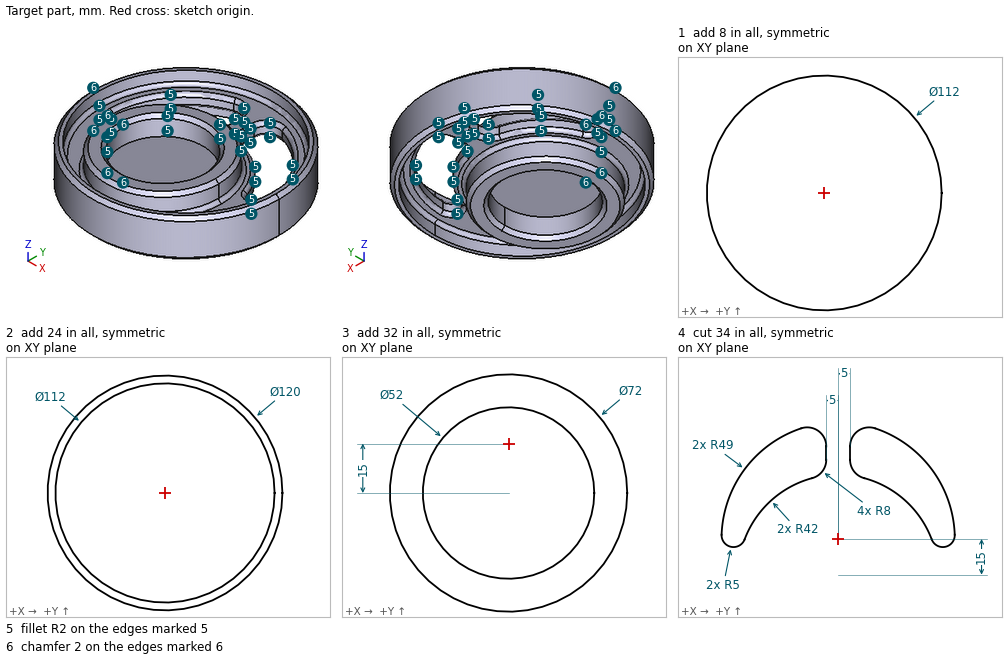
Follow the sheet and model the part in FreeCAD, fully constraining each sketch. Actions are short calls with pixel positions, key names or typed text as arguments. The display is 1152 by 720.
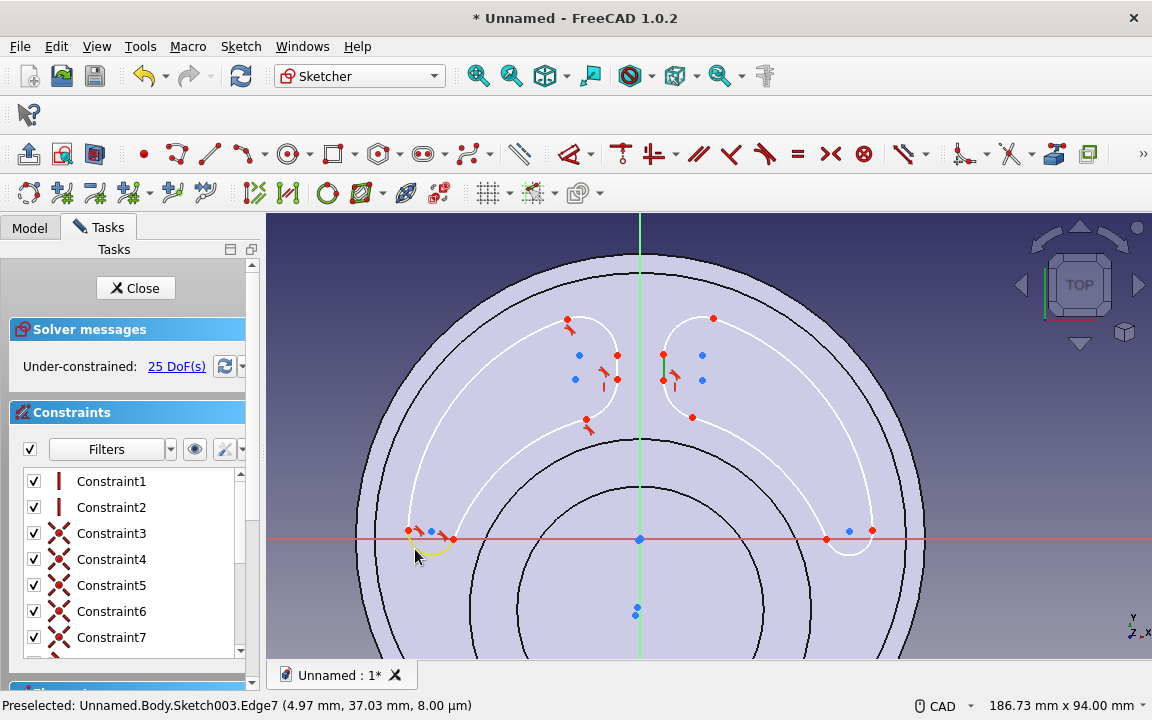
click(693, 318)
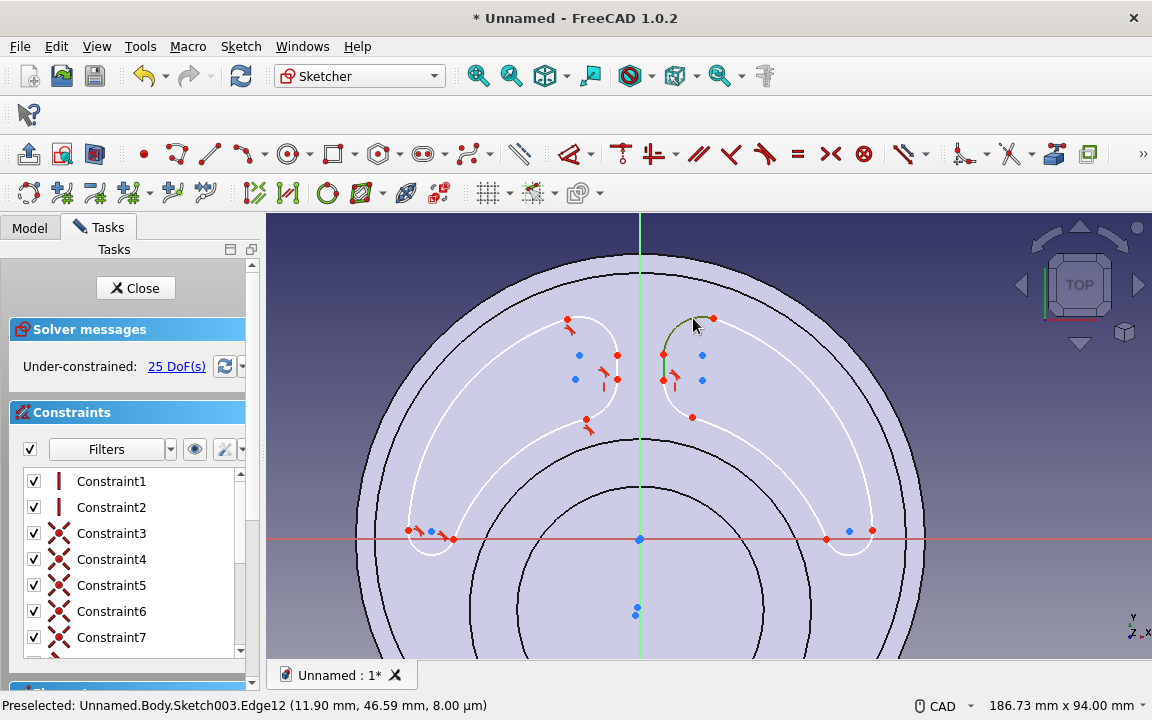
key(t)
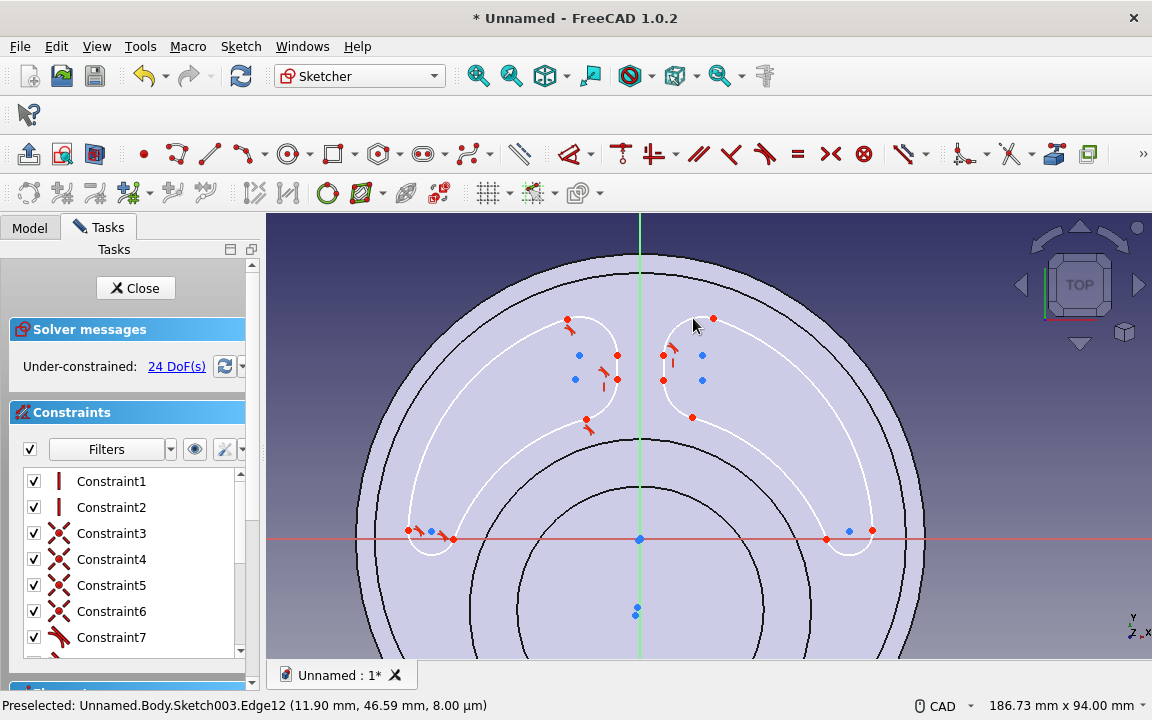
click(667, 395)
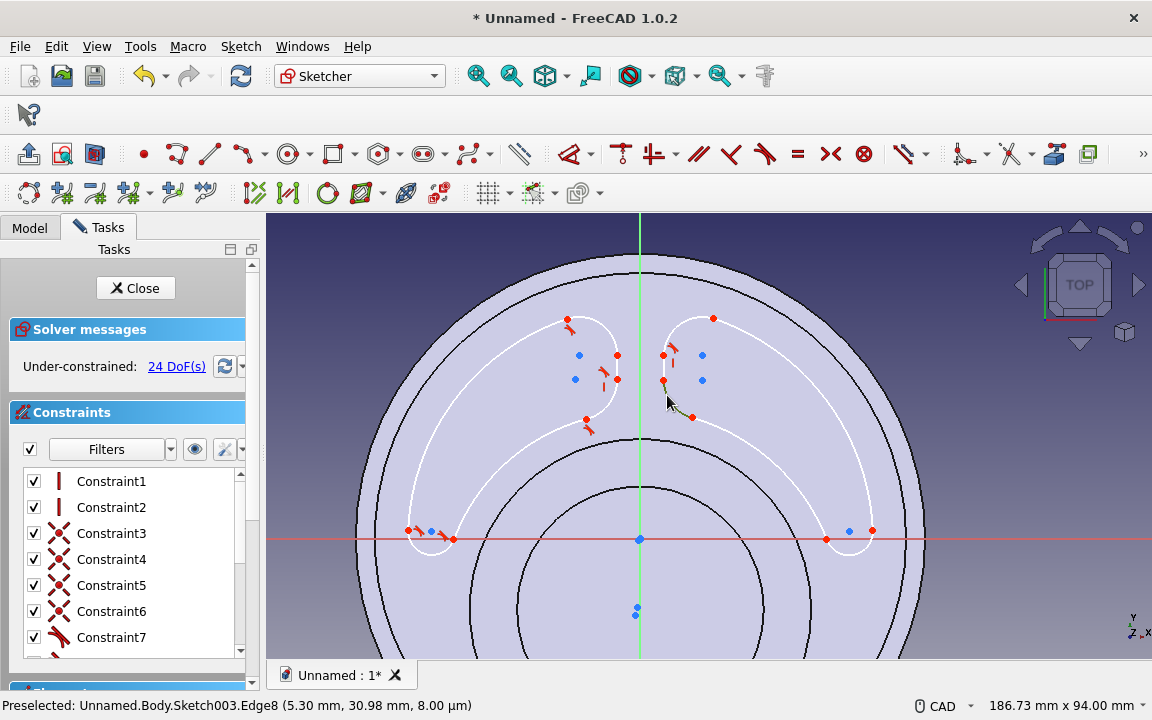
click(799, 491)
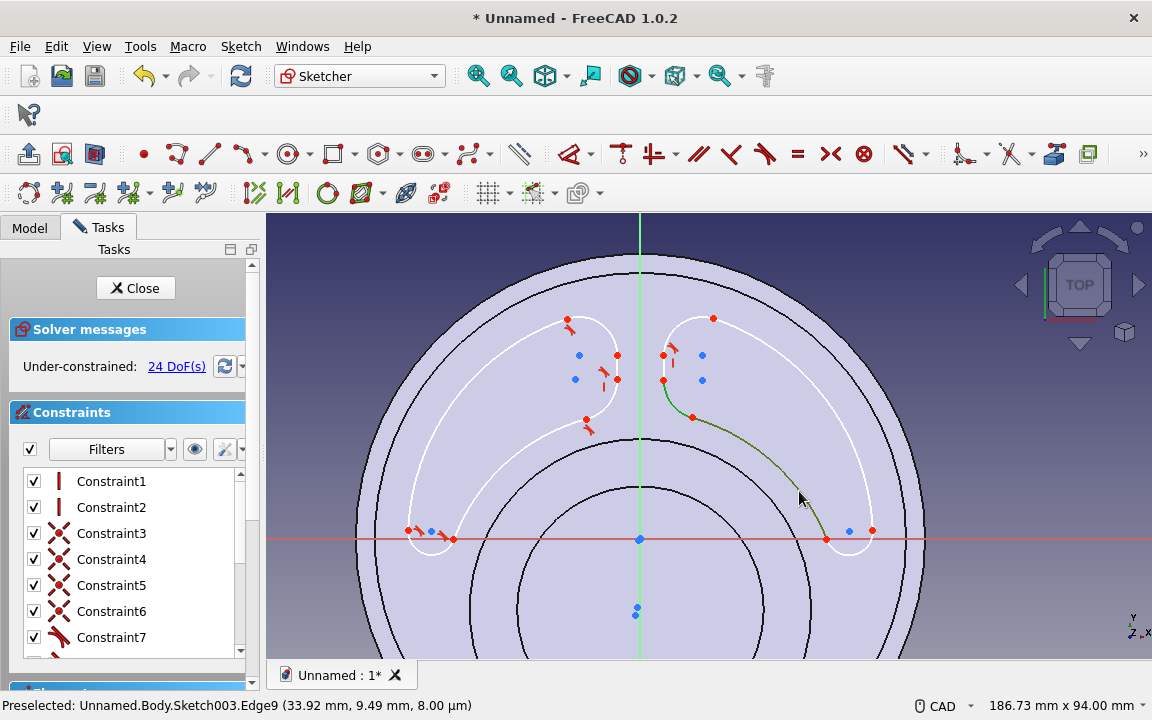
key(t)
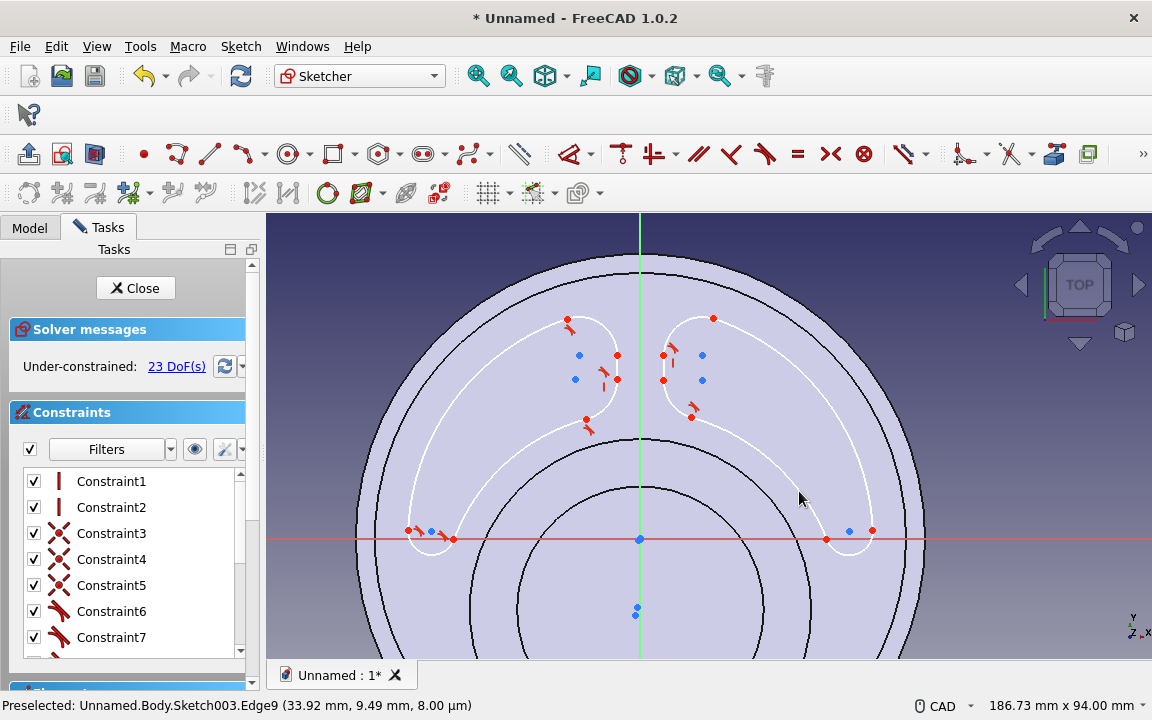
click(799, 490)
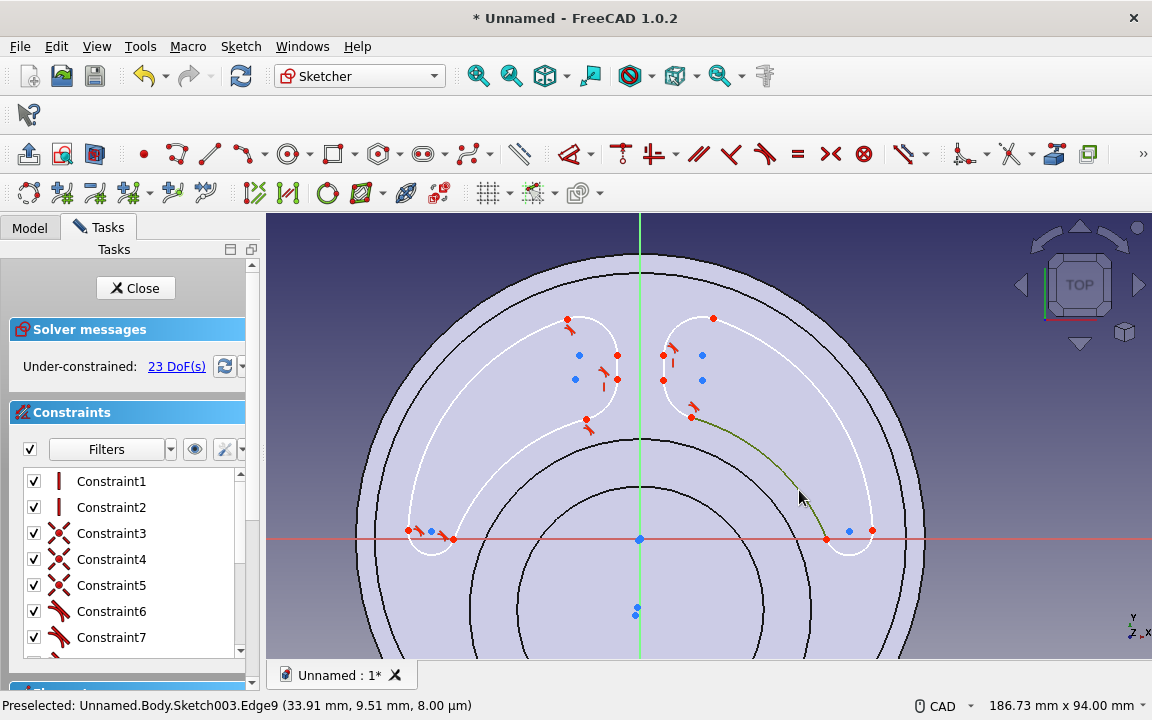
click(840, 554)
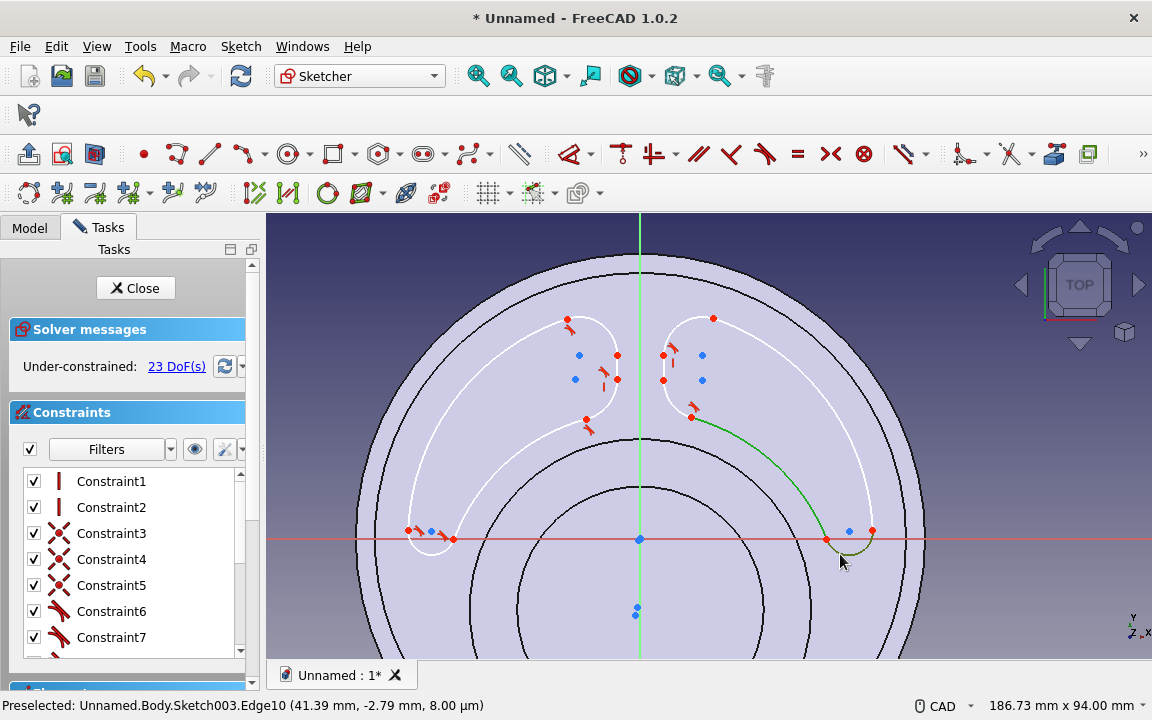
key(t)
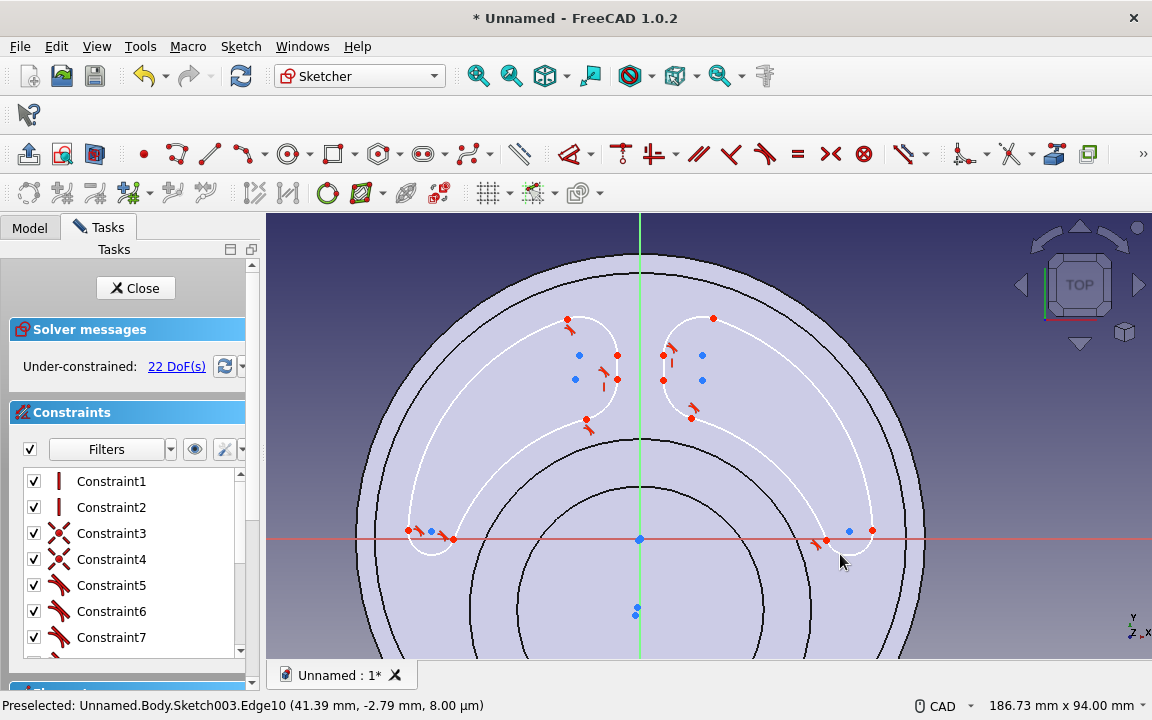
click(841, 554)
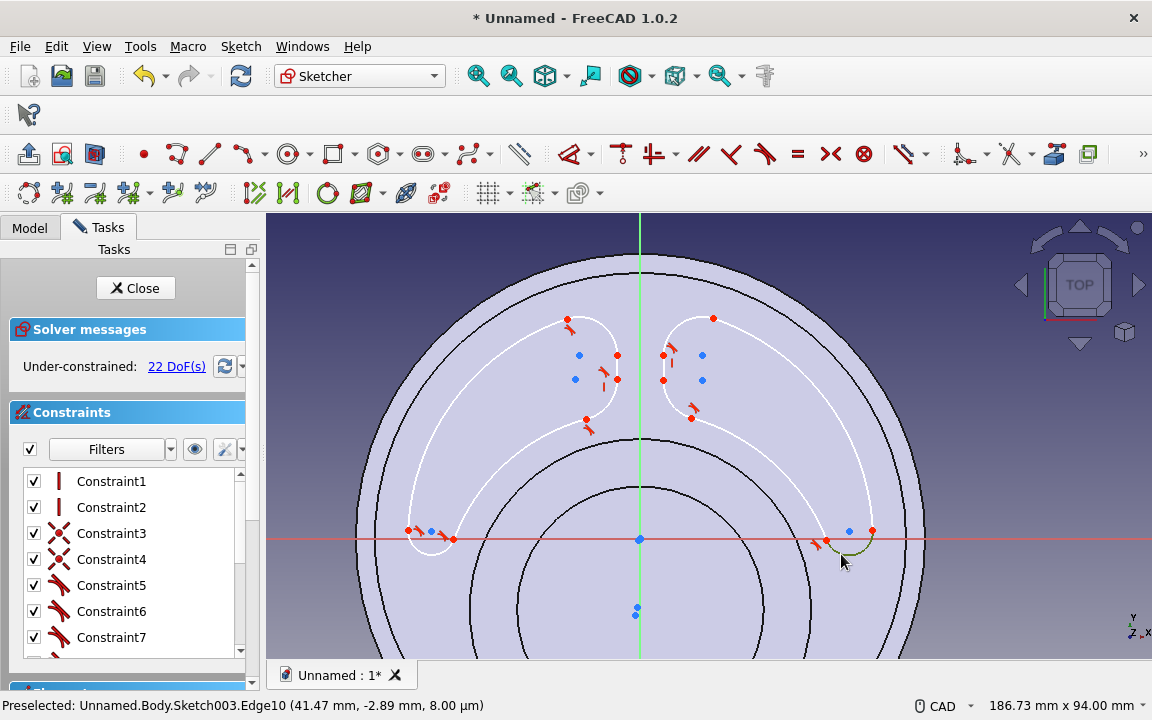
click(854, 449)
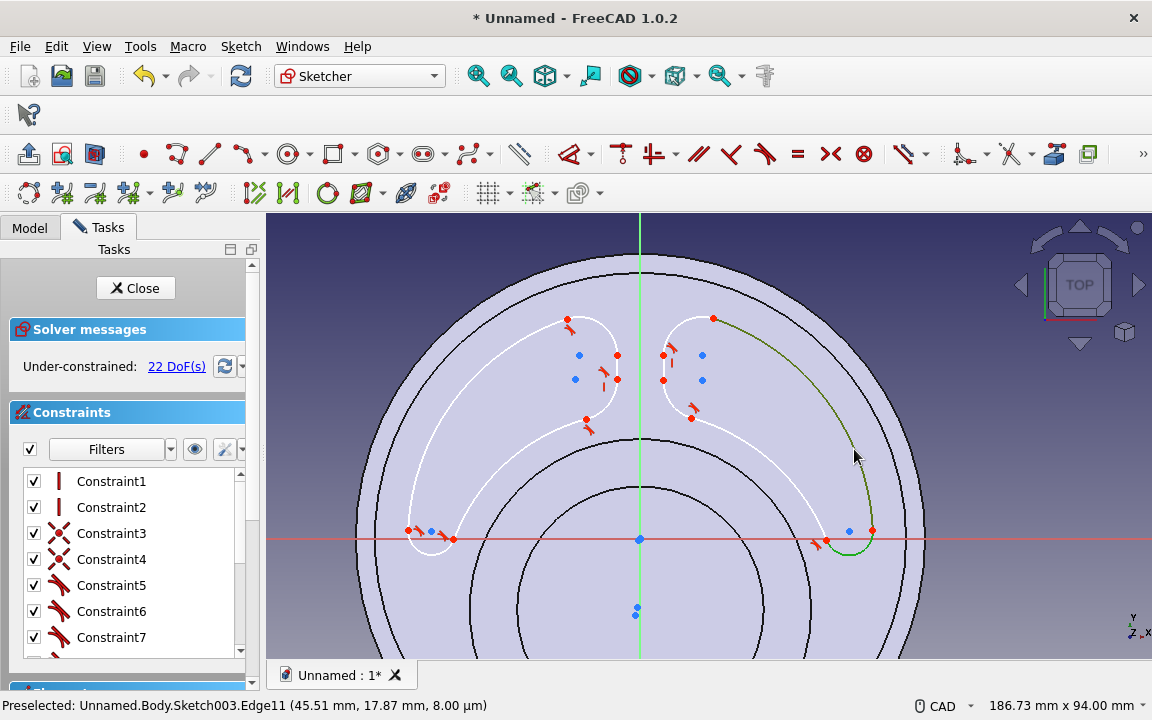
key(t)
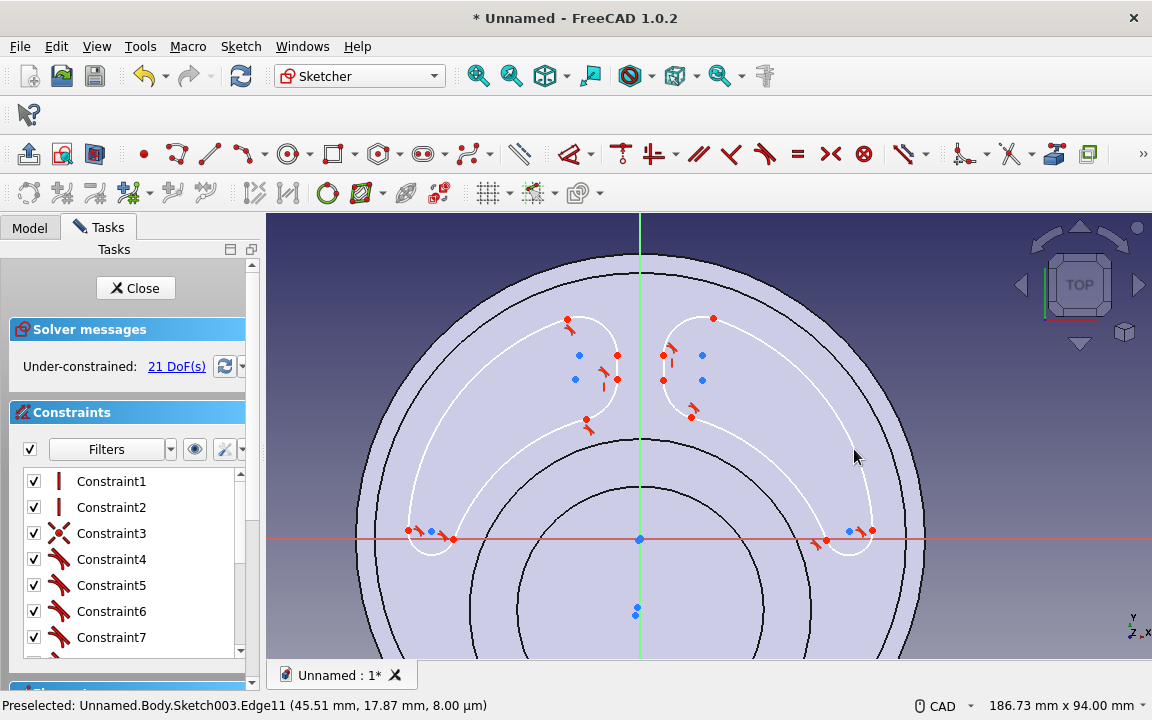
click(854, 449)